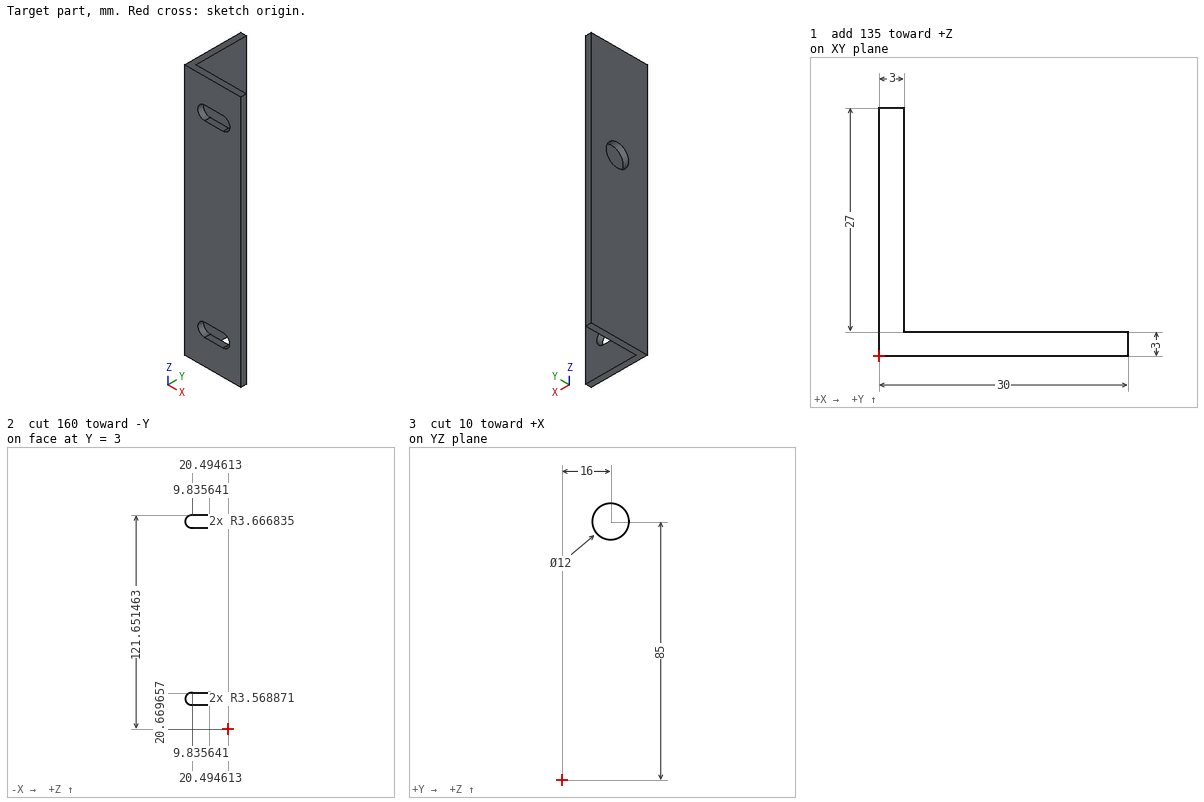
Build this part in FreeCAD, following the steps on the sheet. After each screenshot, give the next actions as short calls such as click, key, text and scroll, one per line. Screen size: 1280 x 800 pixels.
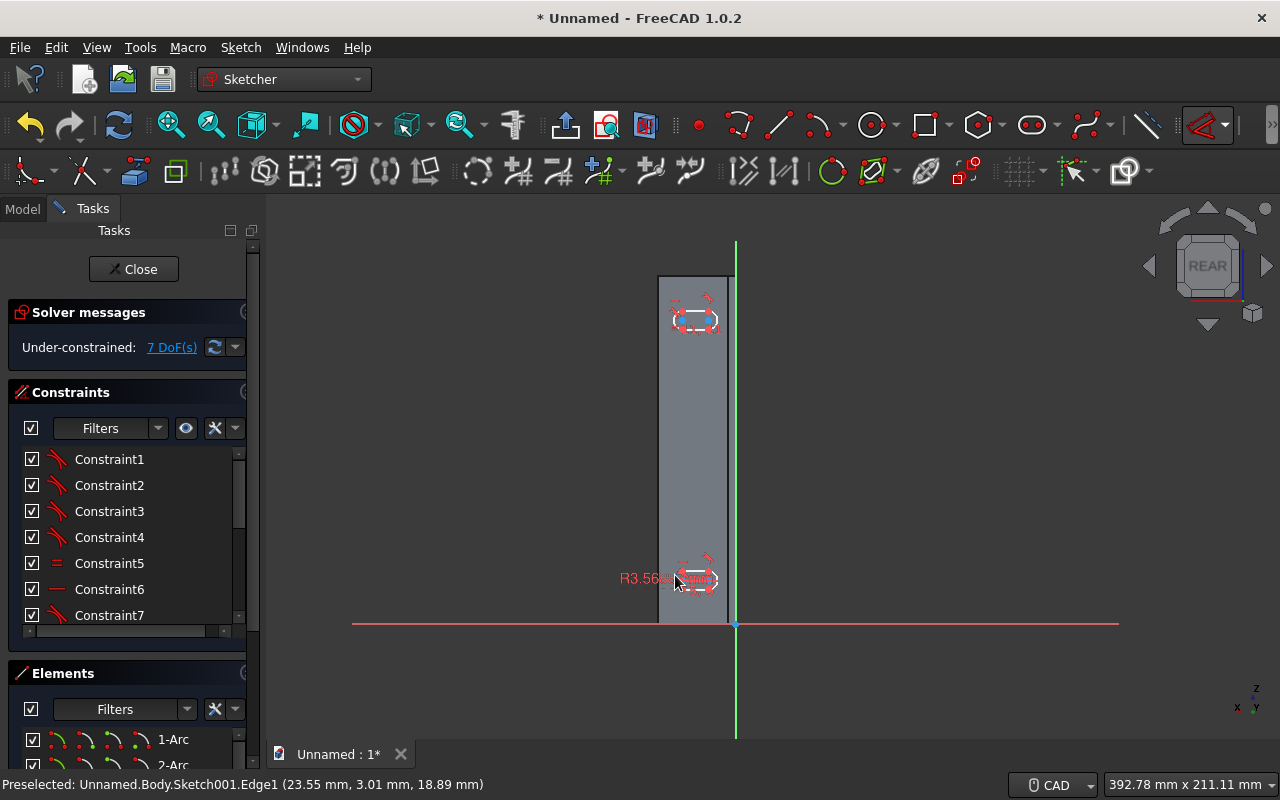
scroll(675, 315, up, 8)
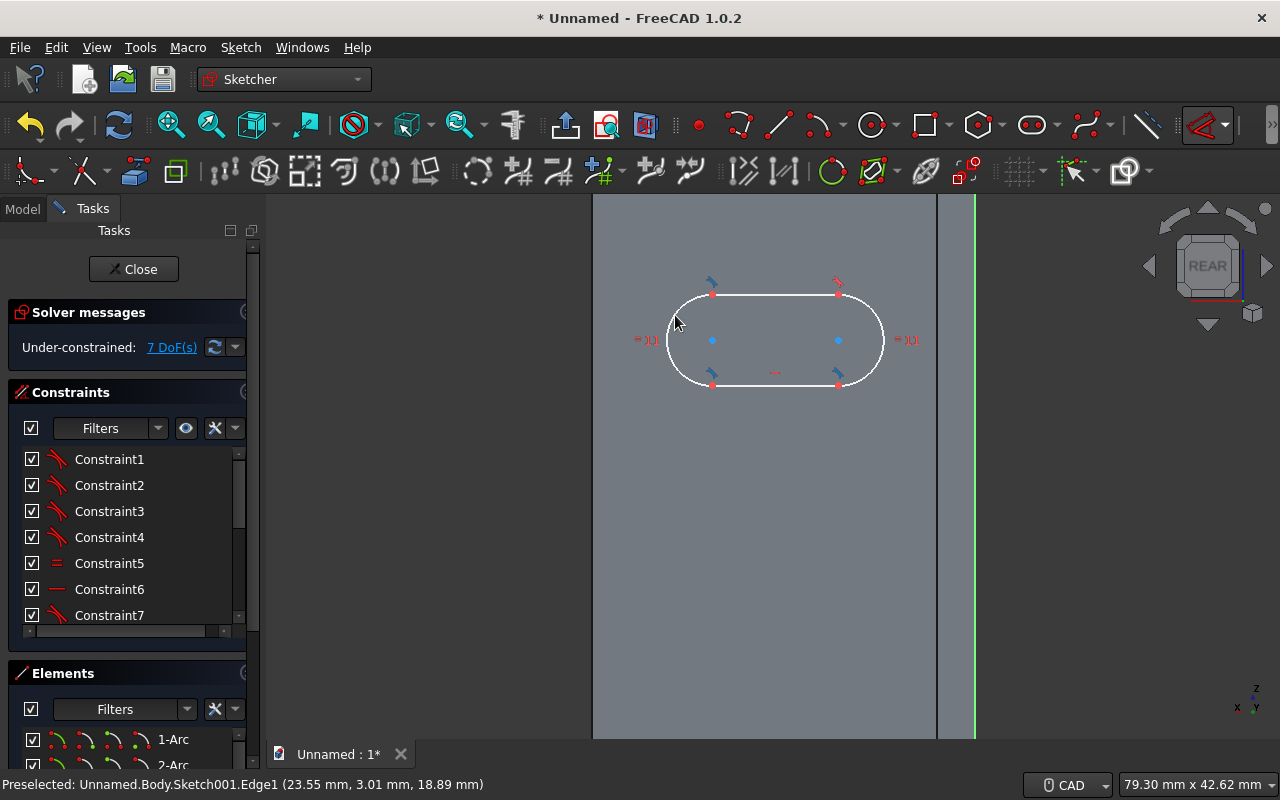
click(676, 314)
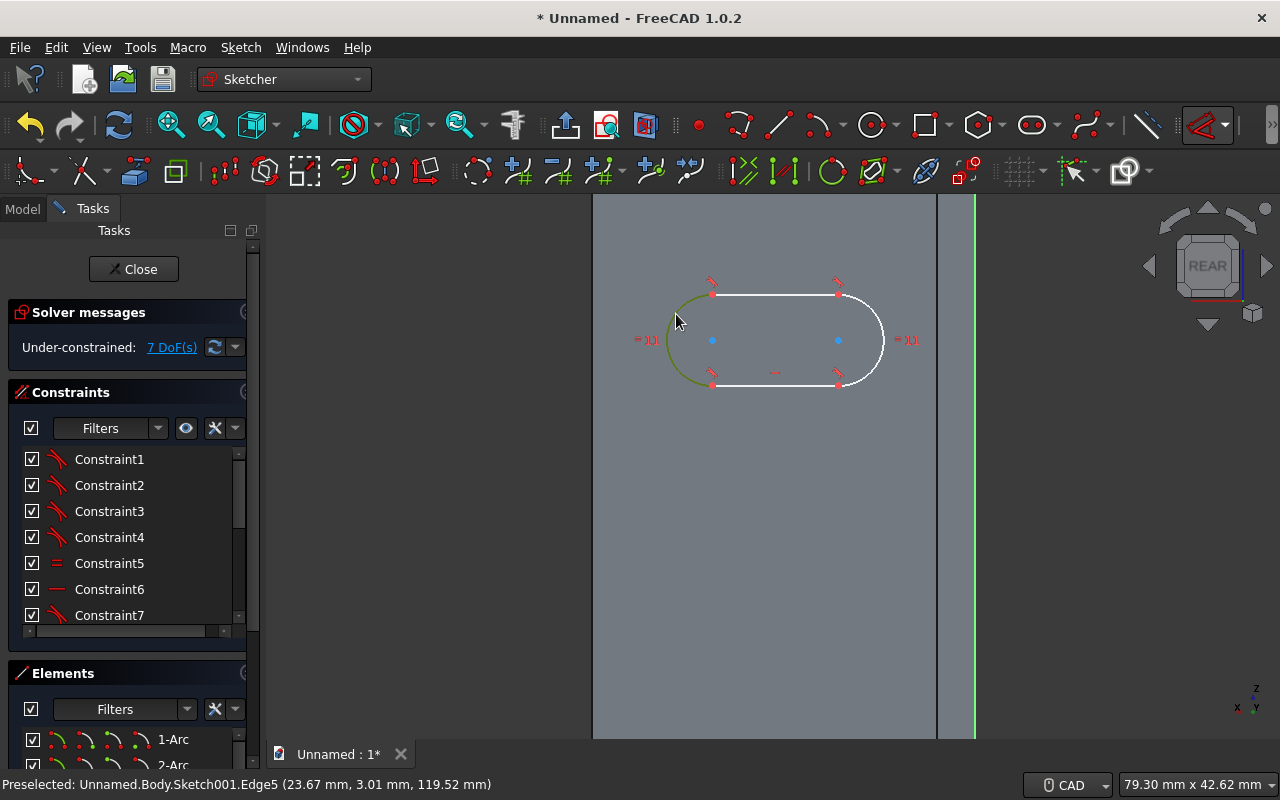
key(k)
key(r)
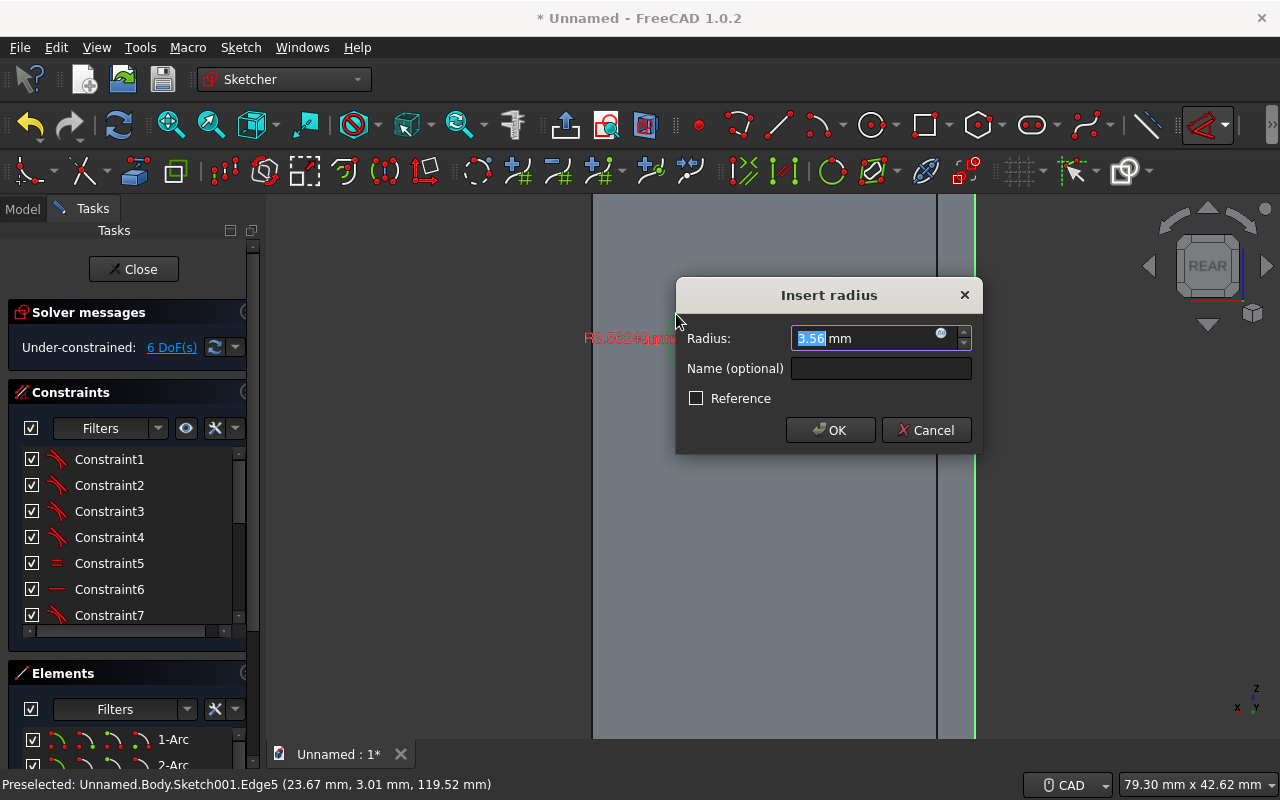
text(3.666835)
key(Return)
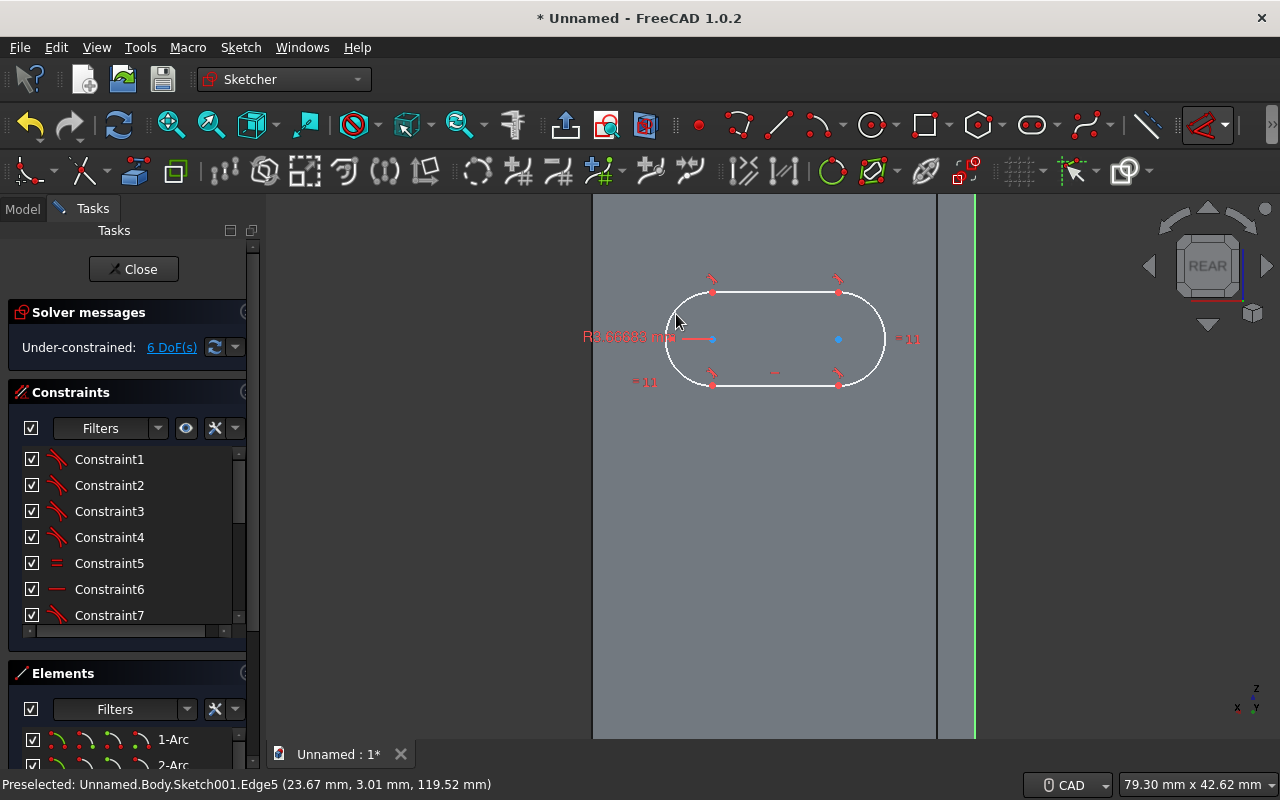
scroll(675, 314, down, 8)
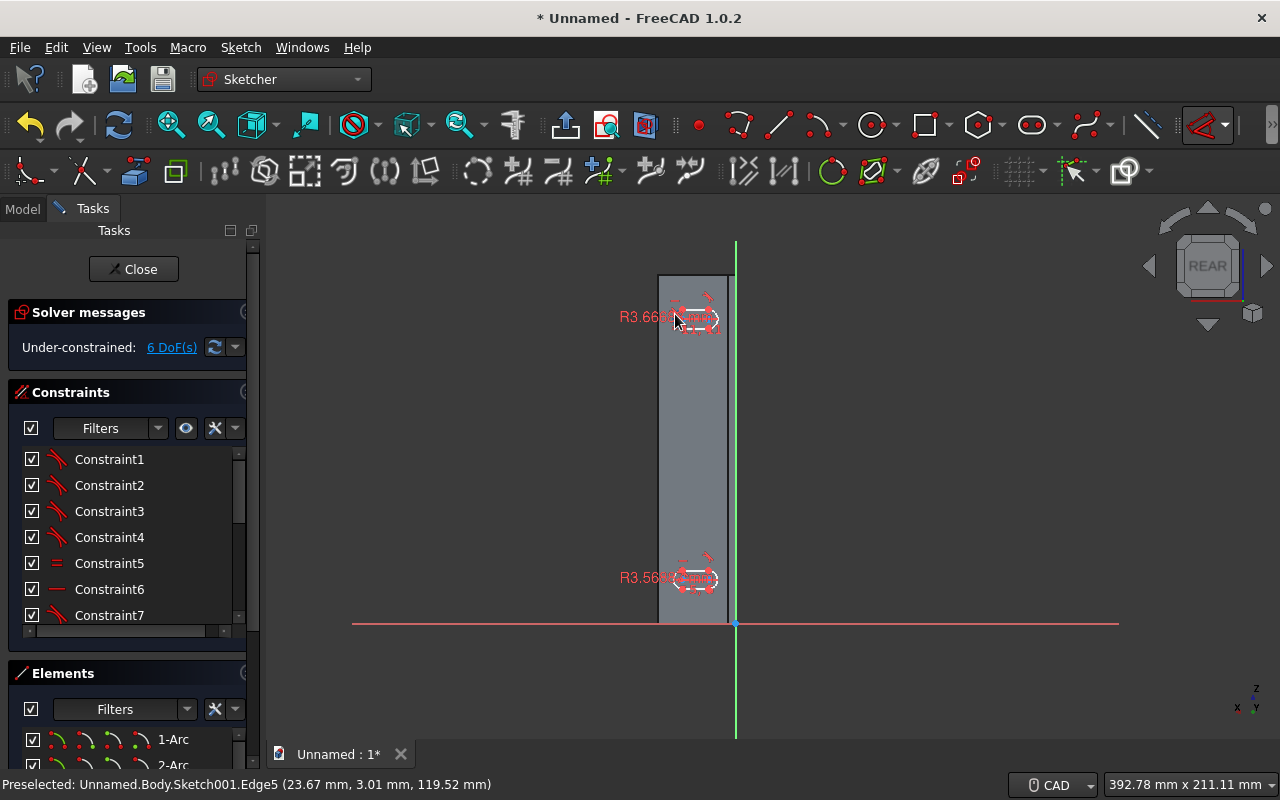
scroll(691, 571, up, 3)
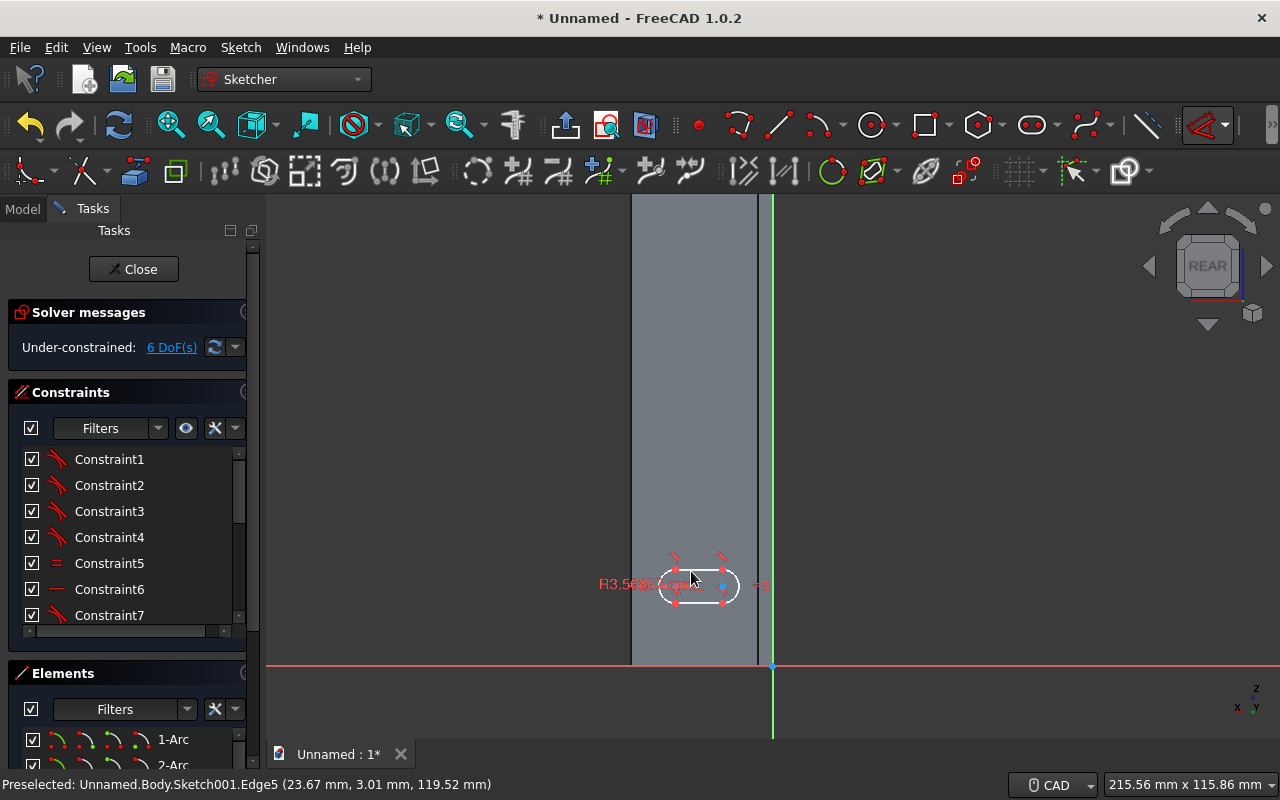
click(690, 570)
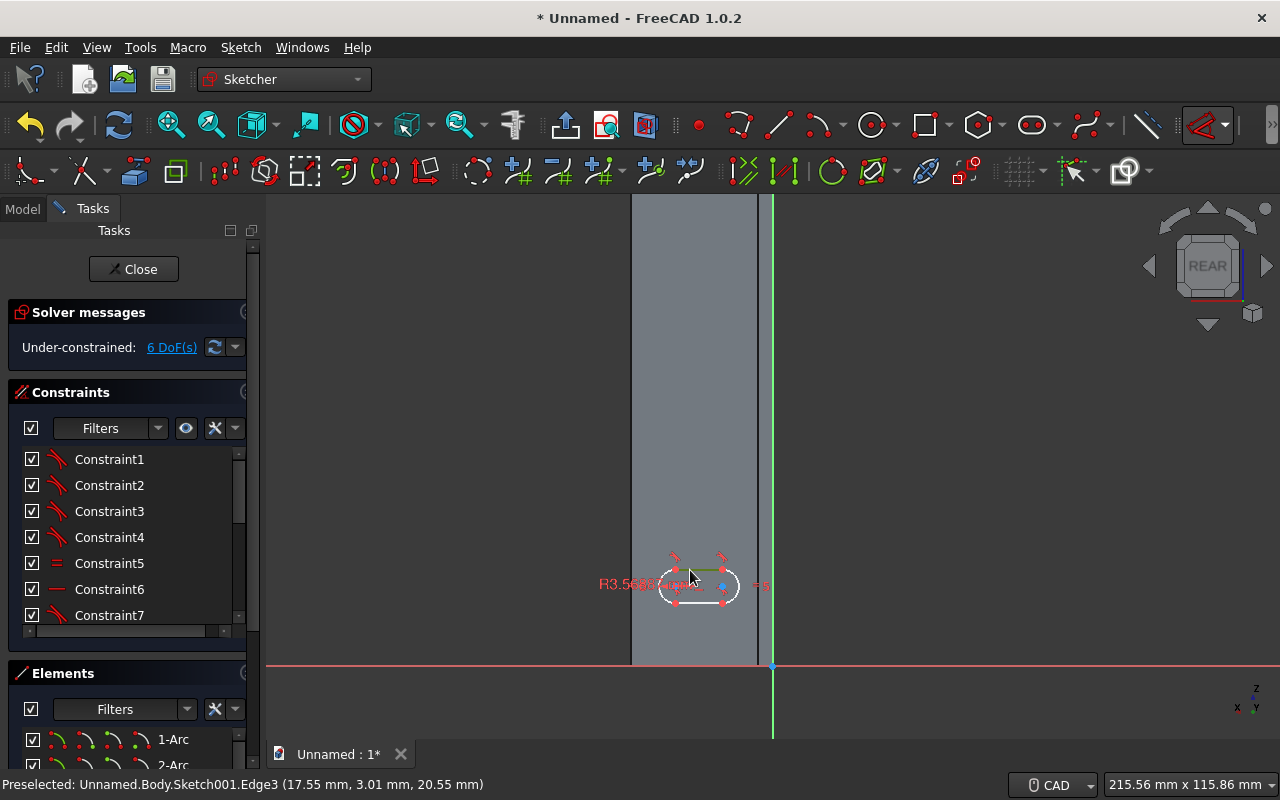
click(1228, 126)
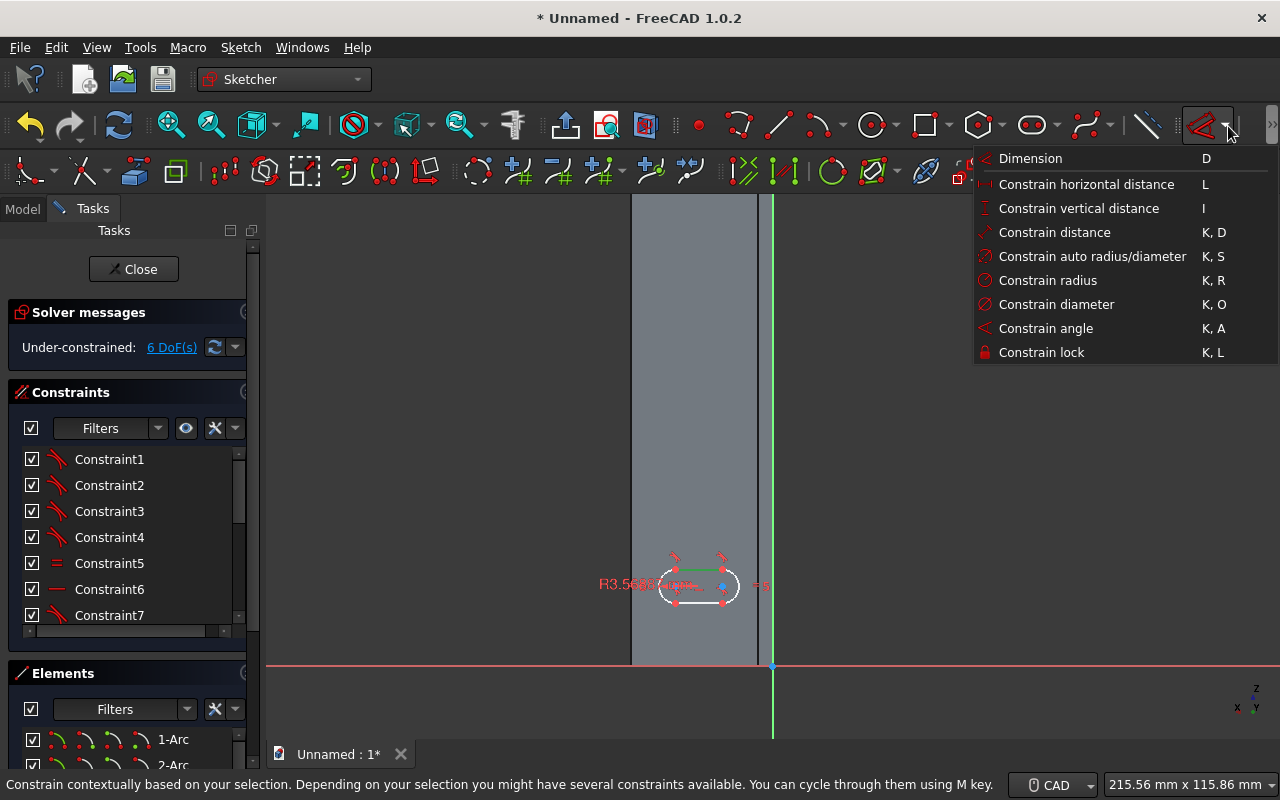
click(1126, 184)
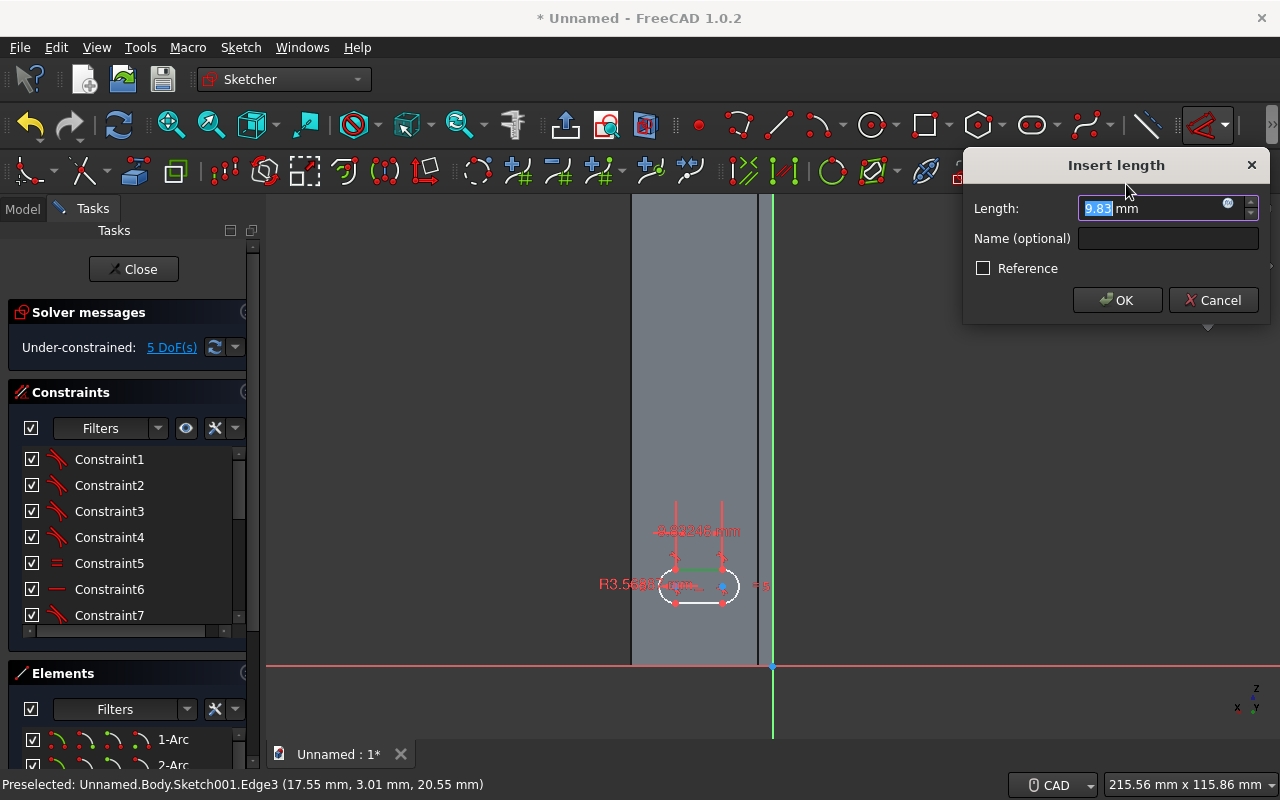
text(9.835641)
key(Return)